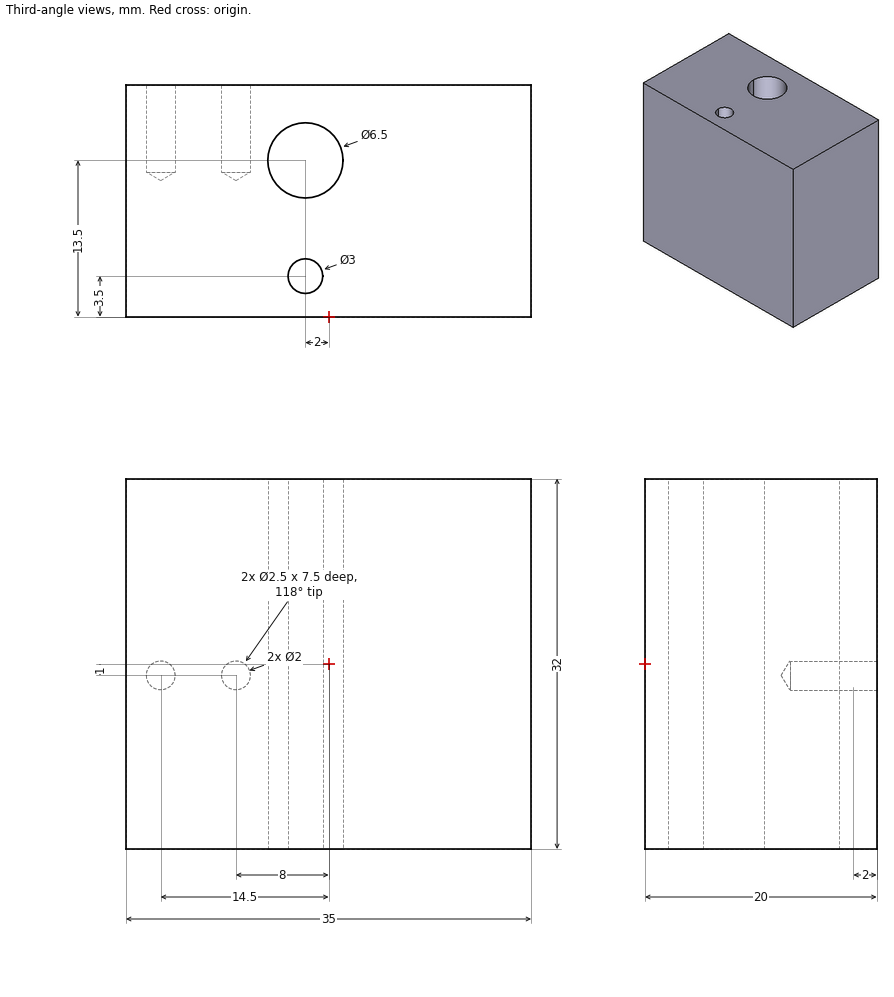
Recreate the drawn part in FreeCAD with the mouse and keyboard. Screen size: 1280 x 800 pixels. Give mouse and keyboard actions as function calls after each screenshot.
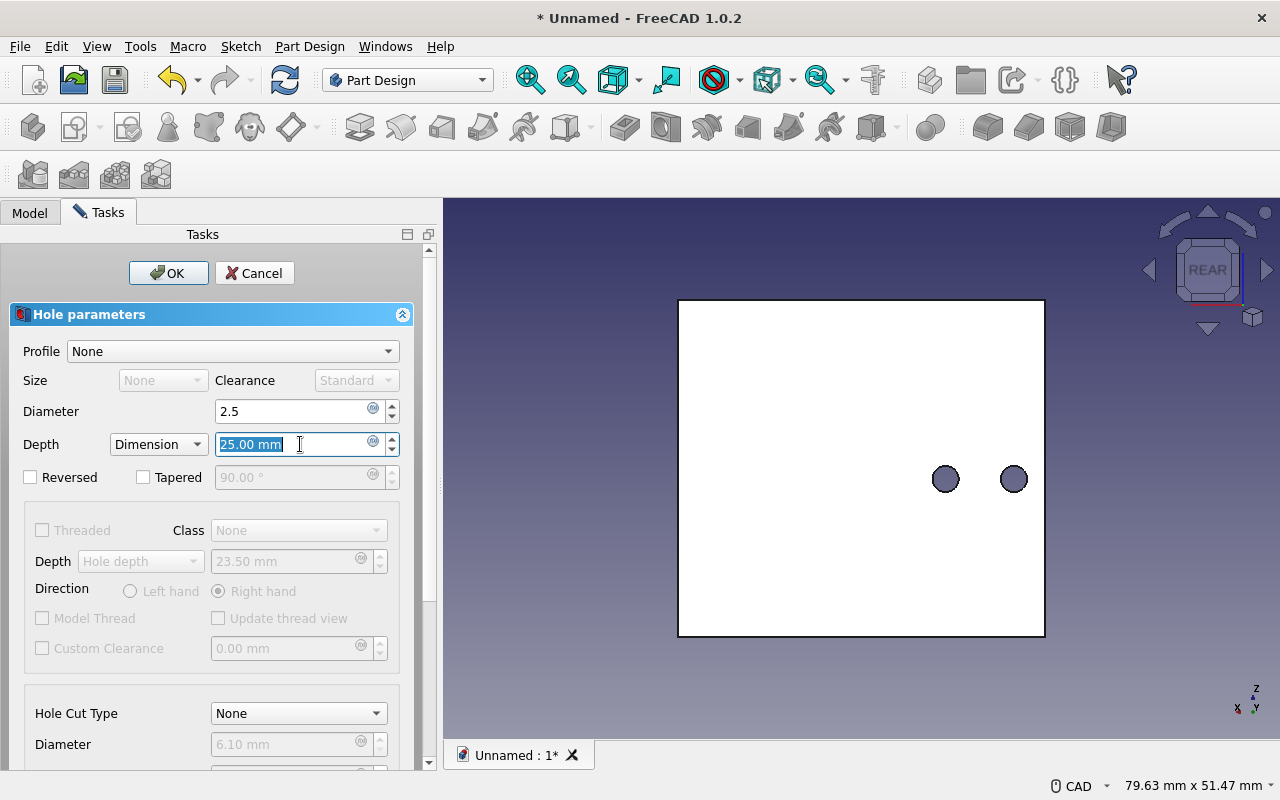
text(7.5)
key(Tab)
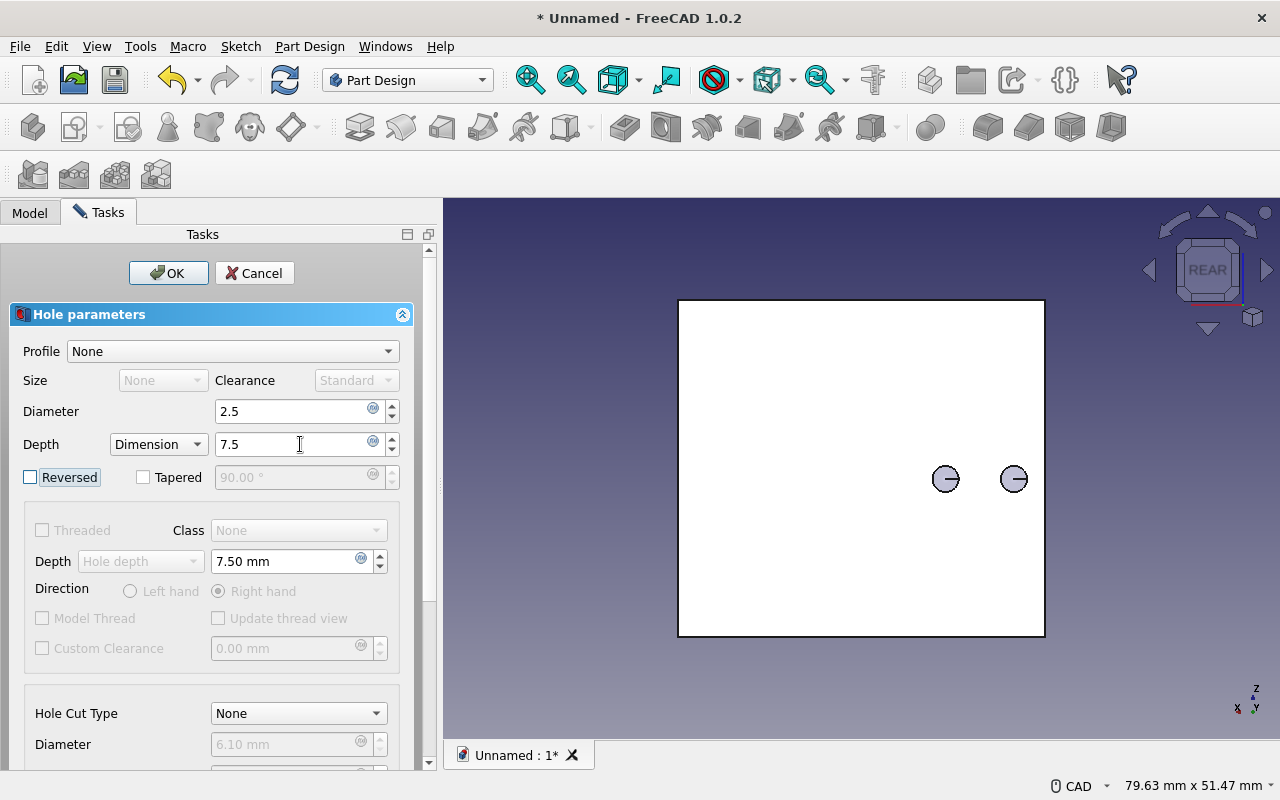
click(169, 273)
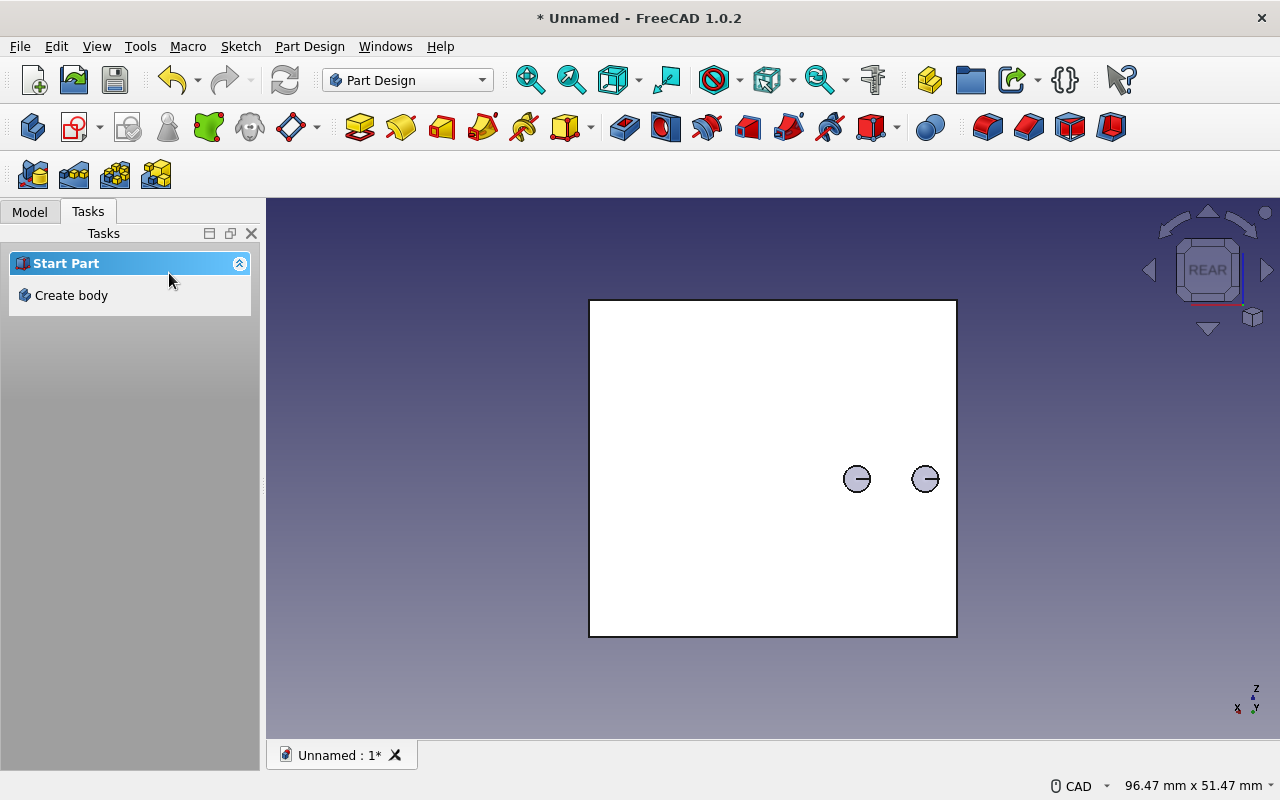
key(0)